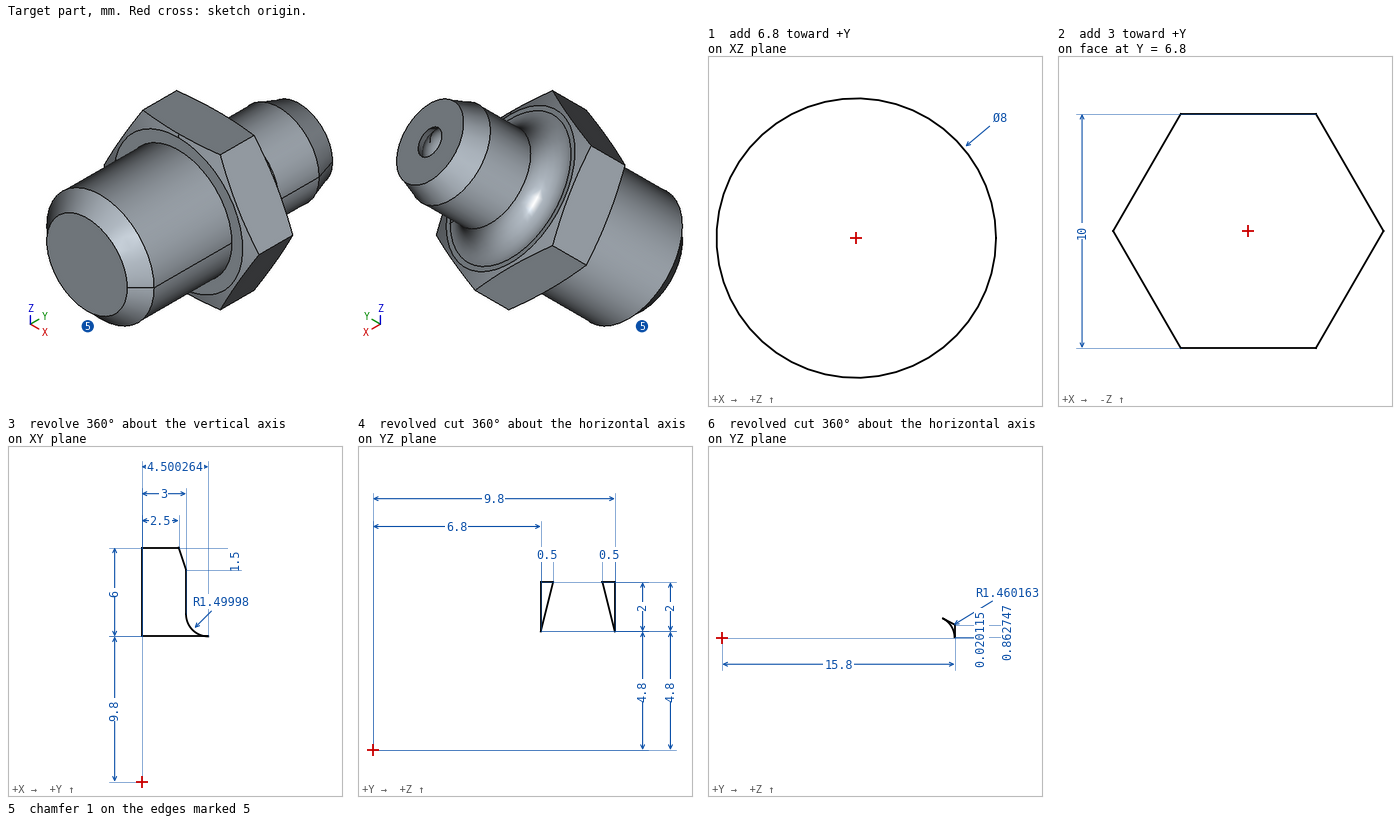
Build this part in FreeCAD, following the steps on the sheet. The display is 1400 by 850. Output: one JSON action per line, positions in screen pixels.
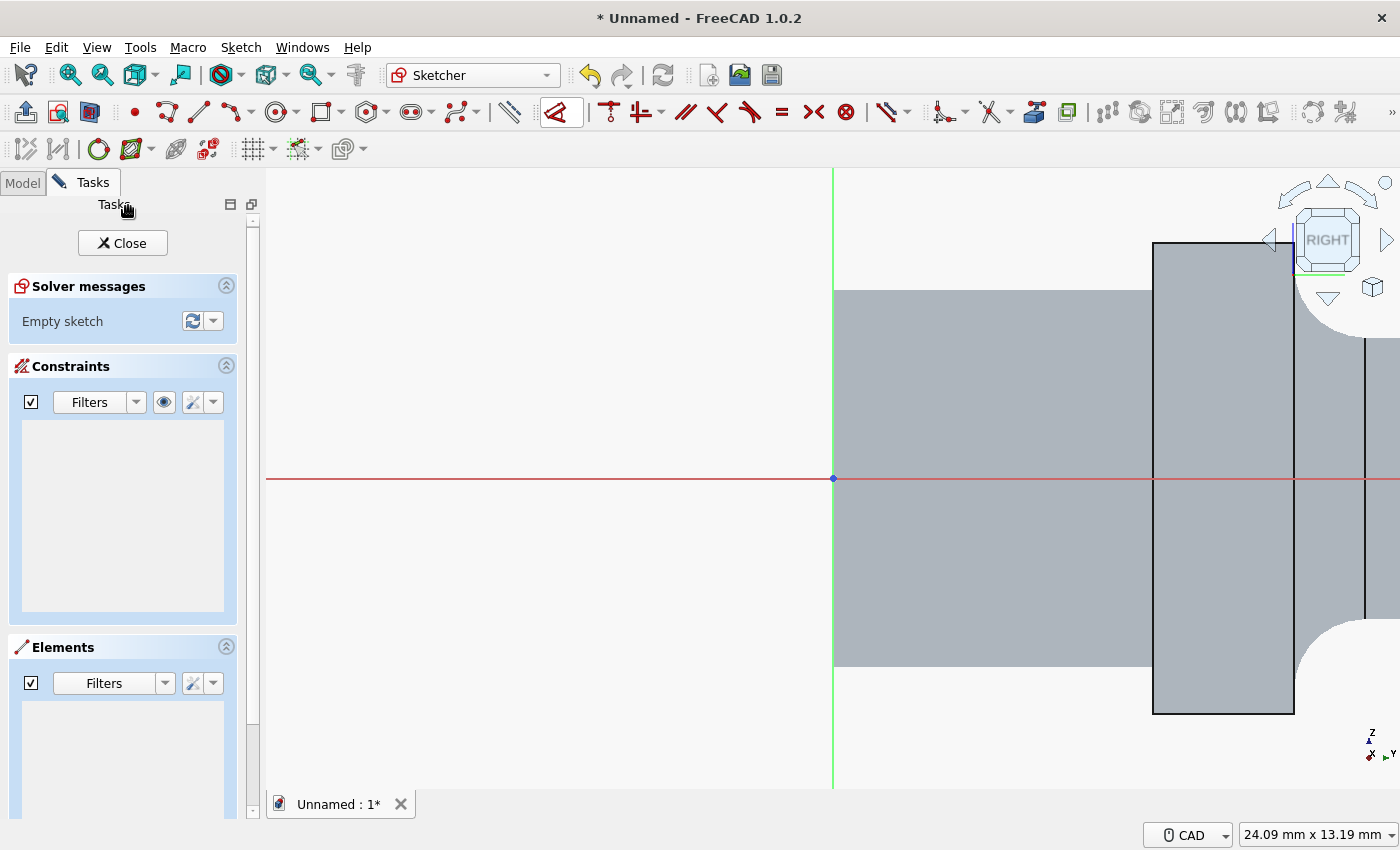
{"action": "scroll", "coordinate": [764, 478], "scroll_direction": "down", "scroll_amount": 5}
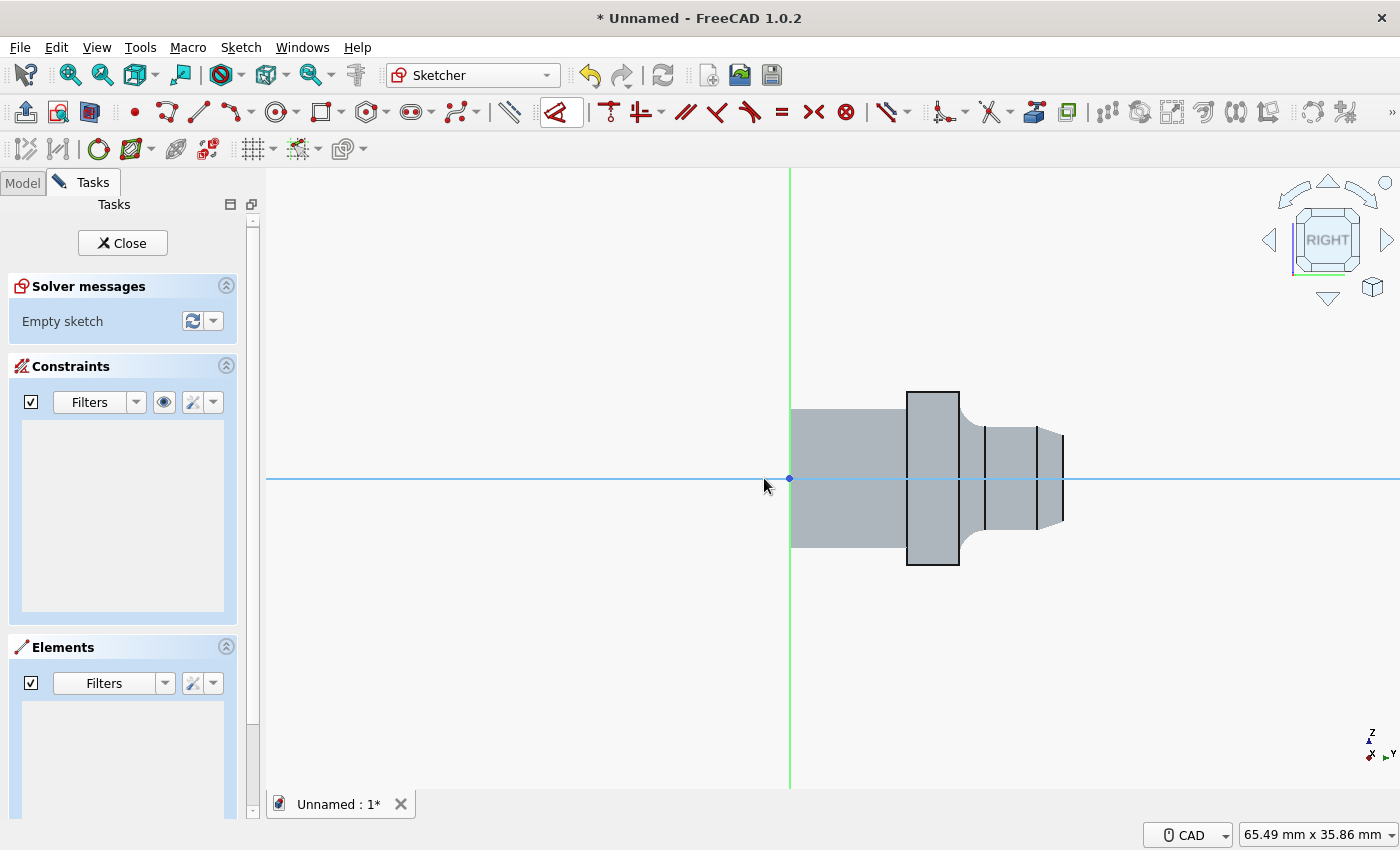
{"action": "scroll", "coordinate": [950, 368], "scroll_direction": "up", "scroll_amount": 12}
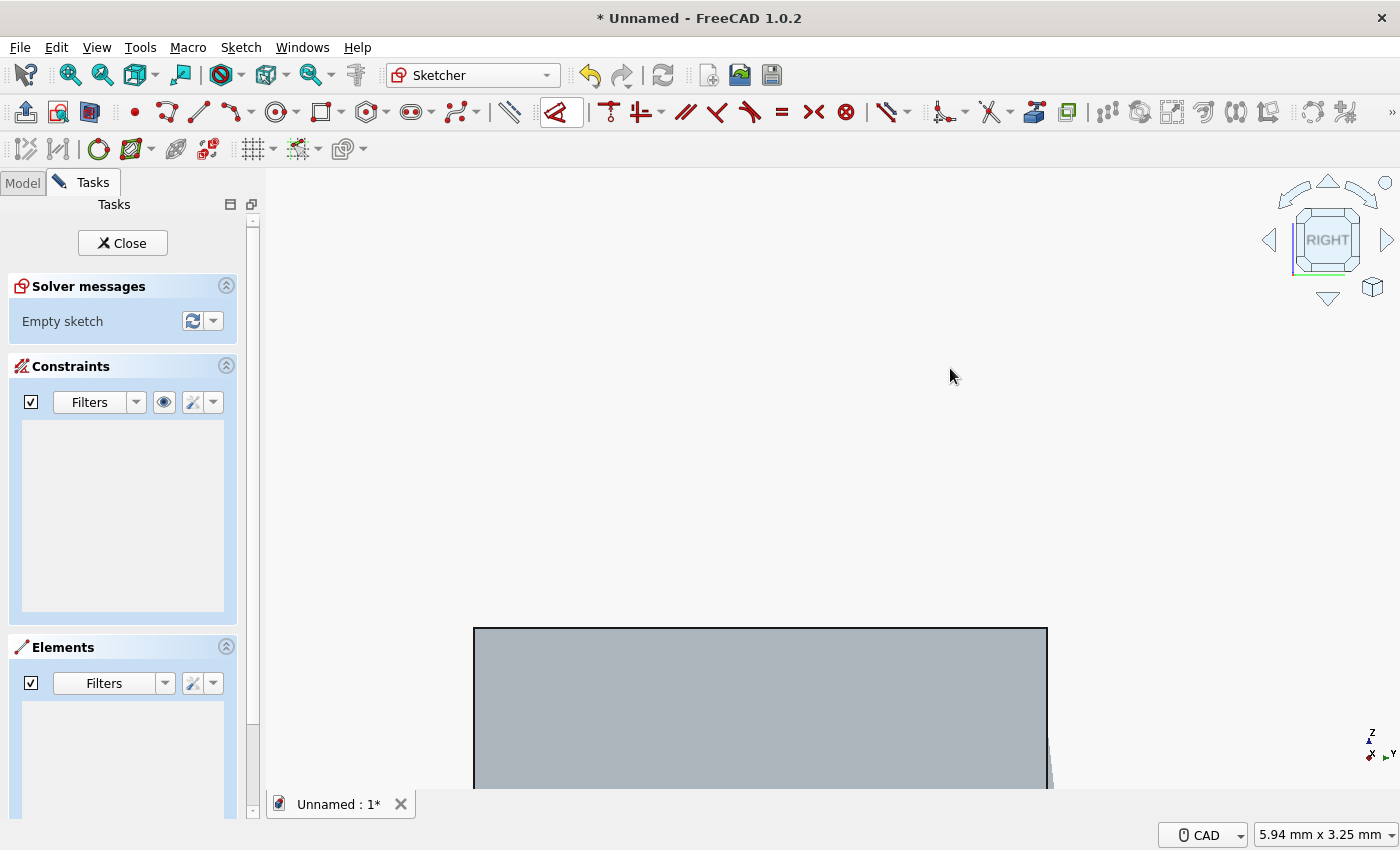
{"action": "key", "text": "g m"}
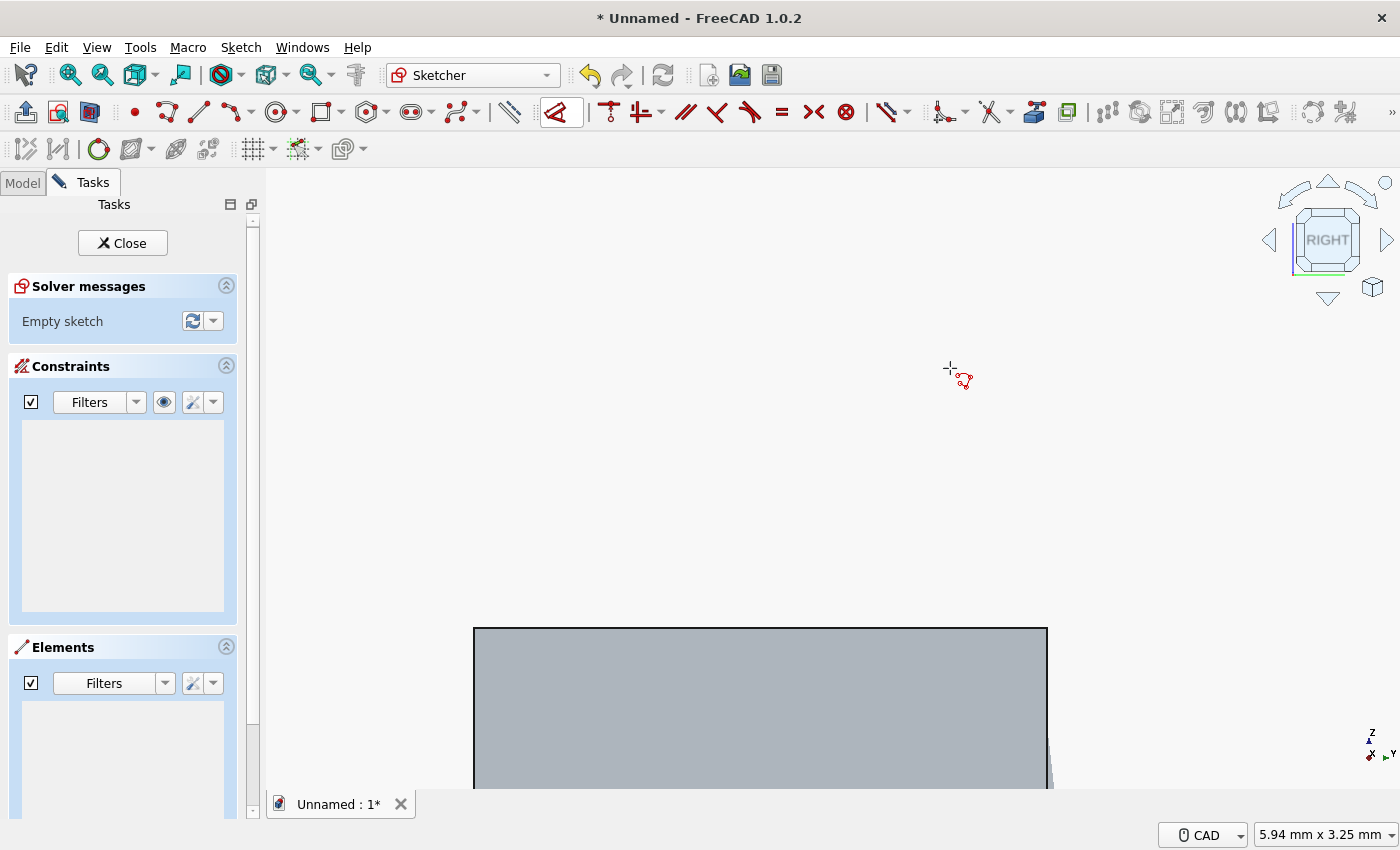
{"action": "left_click", "coordinate": [1047, 667]}
{"action": "left_click", "coordinate": [1047, 285]}
{"action": "left_click", "coordinate": [952, 285]}
{"action": "left_click", "coordinate": [1047, 668]}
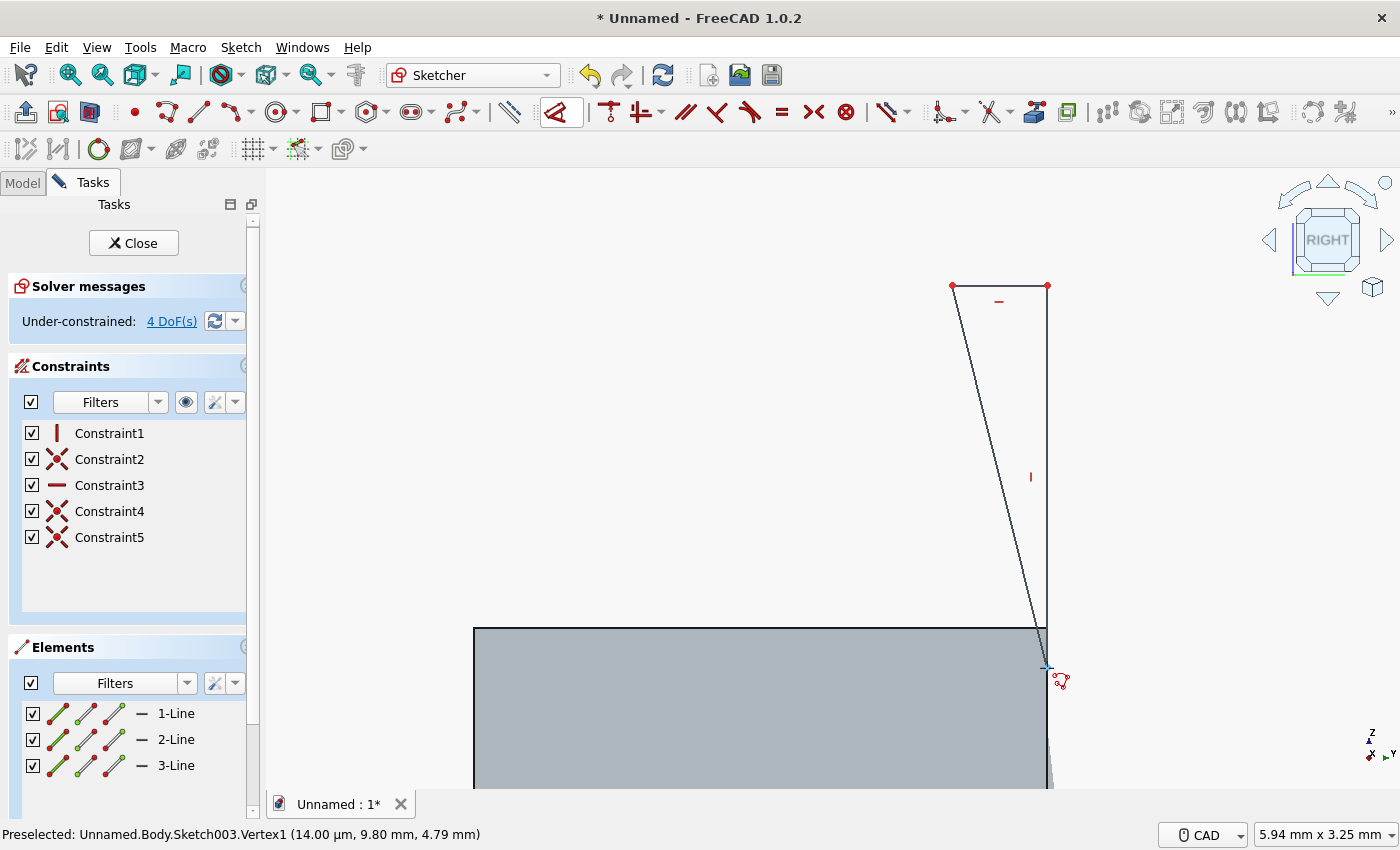
{"action": "left_click", "coordinate": [474, 667]}
{"action": "left_click", "coordinate": [570, 285]}
{"action": "left_click", "coordinate": [474, 285]}
{"action": "left_click", "coordinate": [474, 668]}
{"action": "key", "text": "Escape"}
{"action": "key", "text": "Escape"}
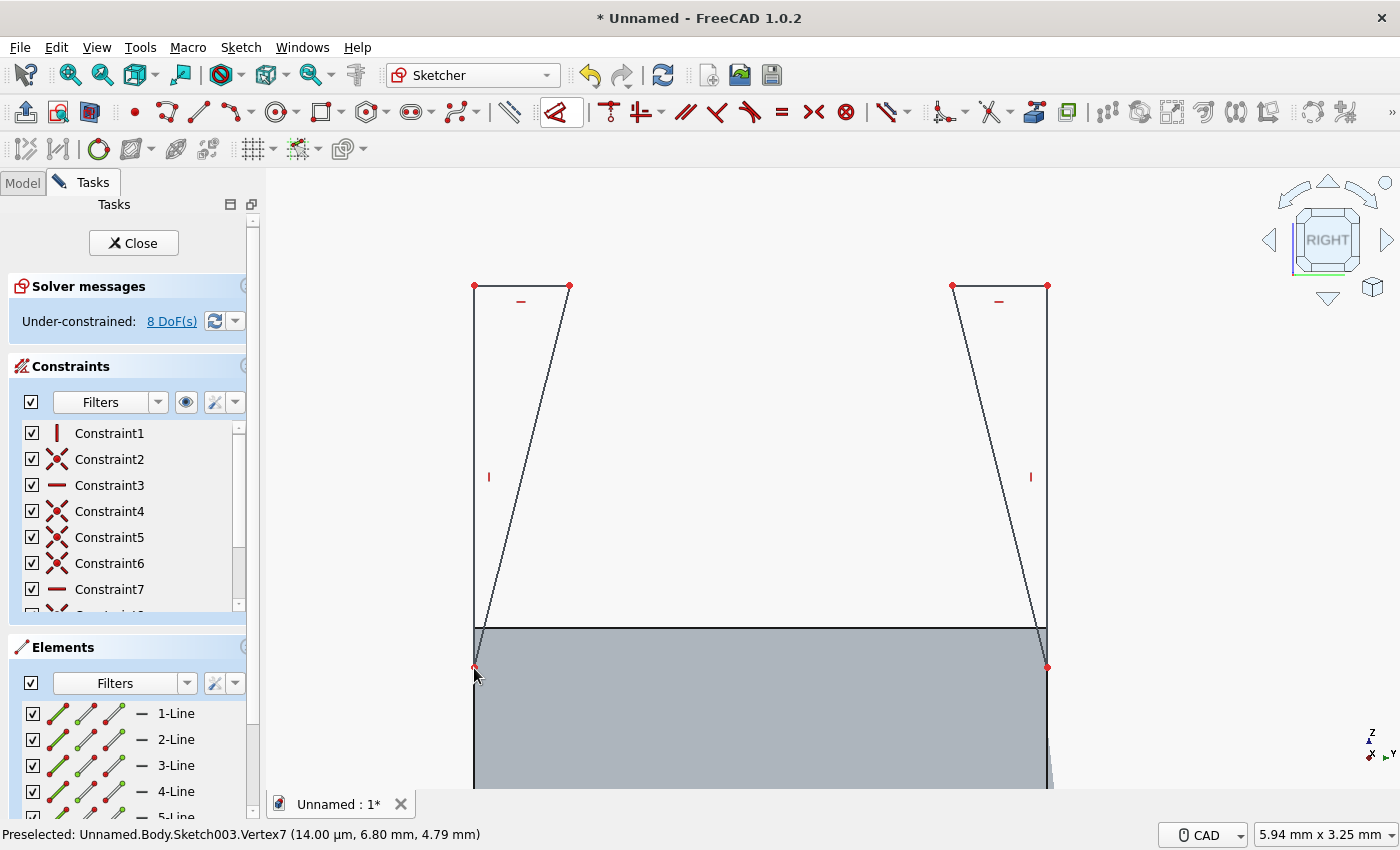
{"action": "left_click", "coordinate": [1047, 553]}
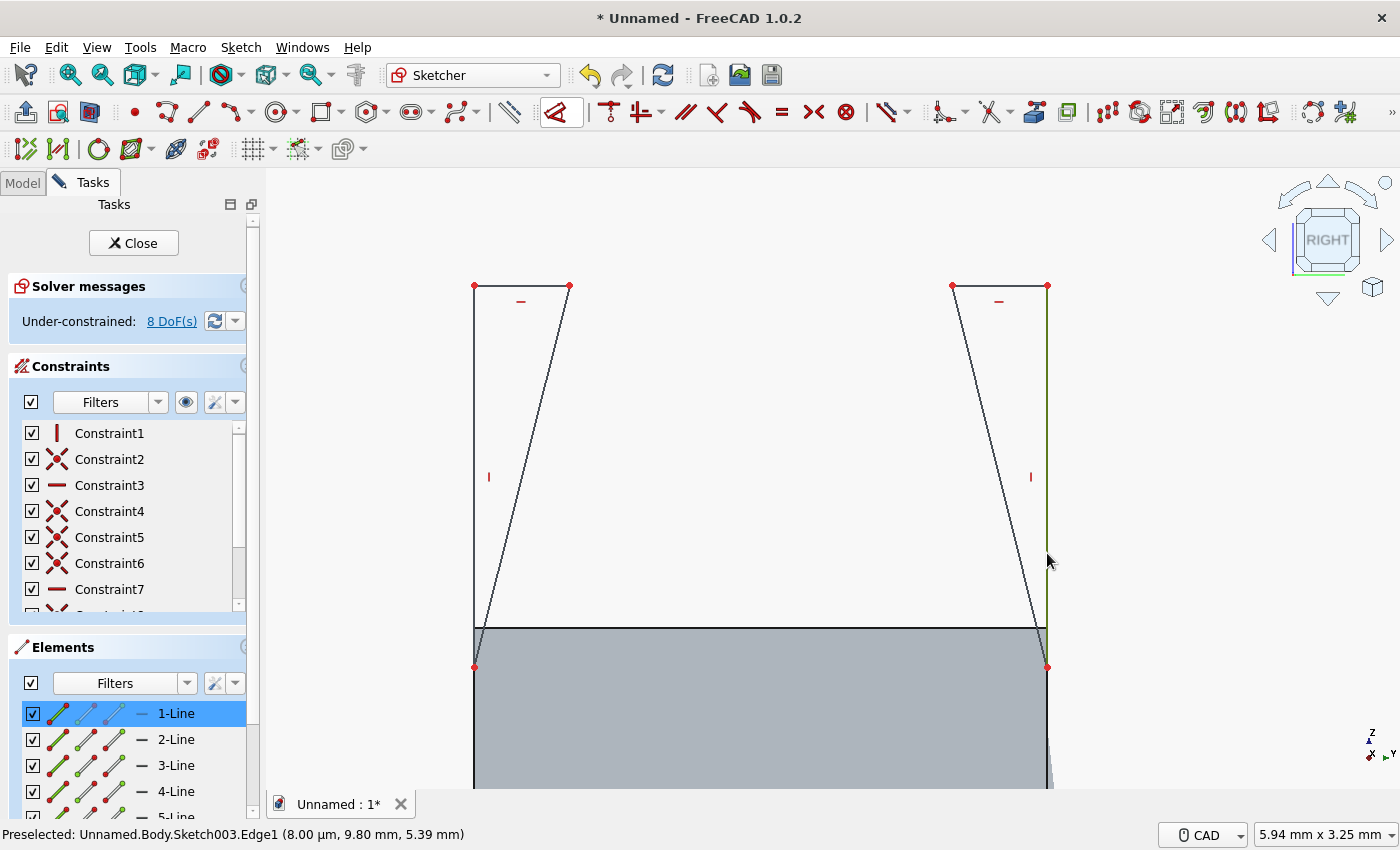
{"action": "left_click", "coordinate": [578, 112]}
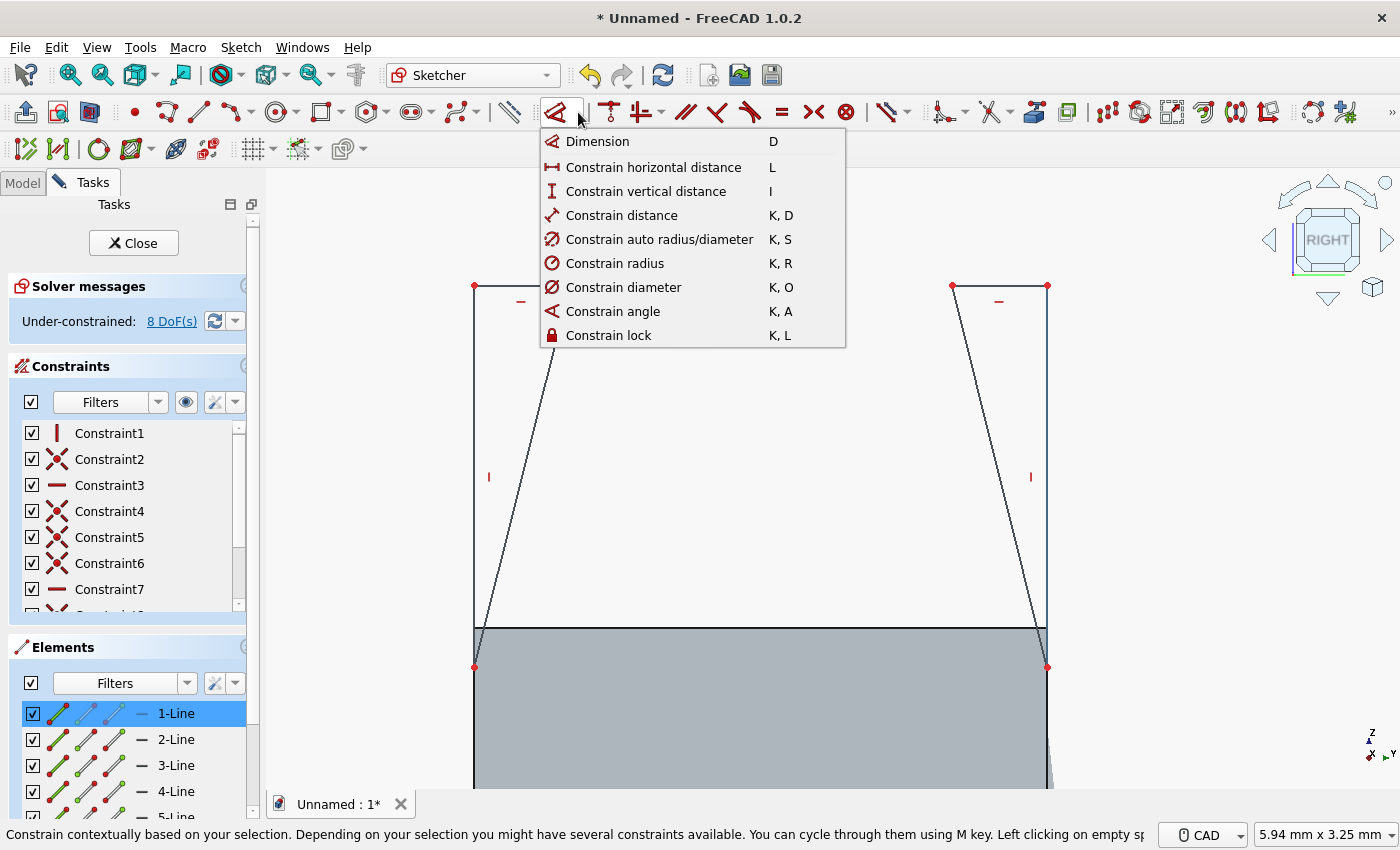
{"action": "left_click", "coordinate": [693, 191]}